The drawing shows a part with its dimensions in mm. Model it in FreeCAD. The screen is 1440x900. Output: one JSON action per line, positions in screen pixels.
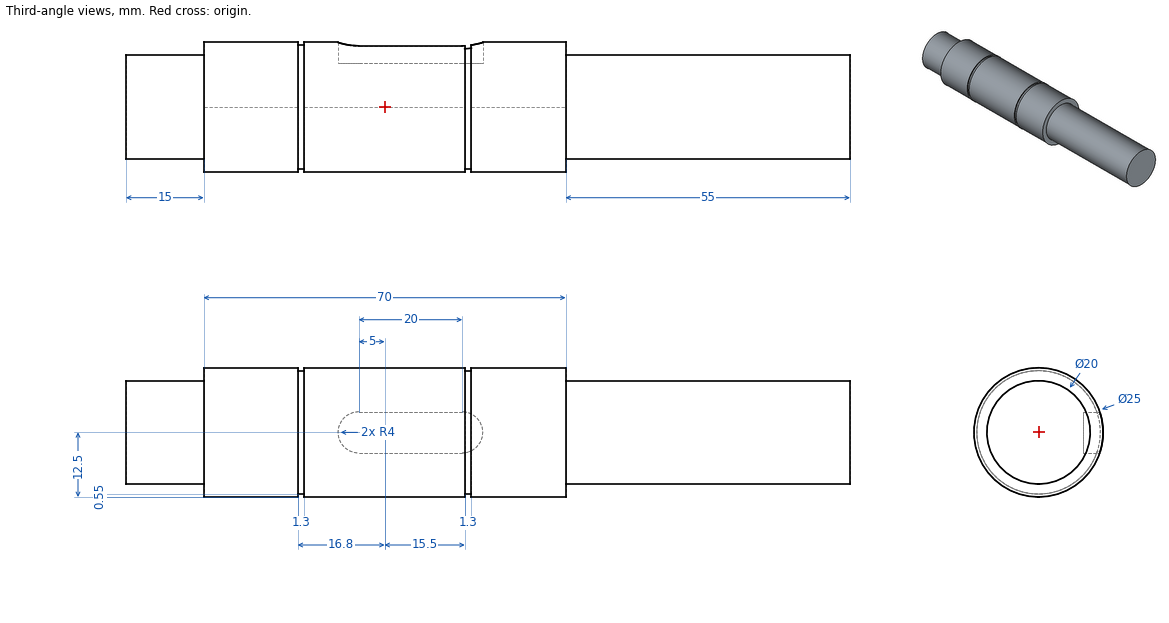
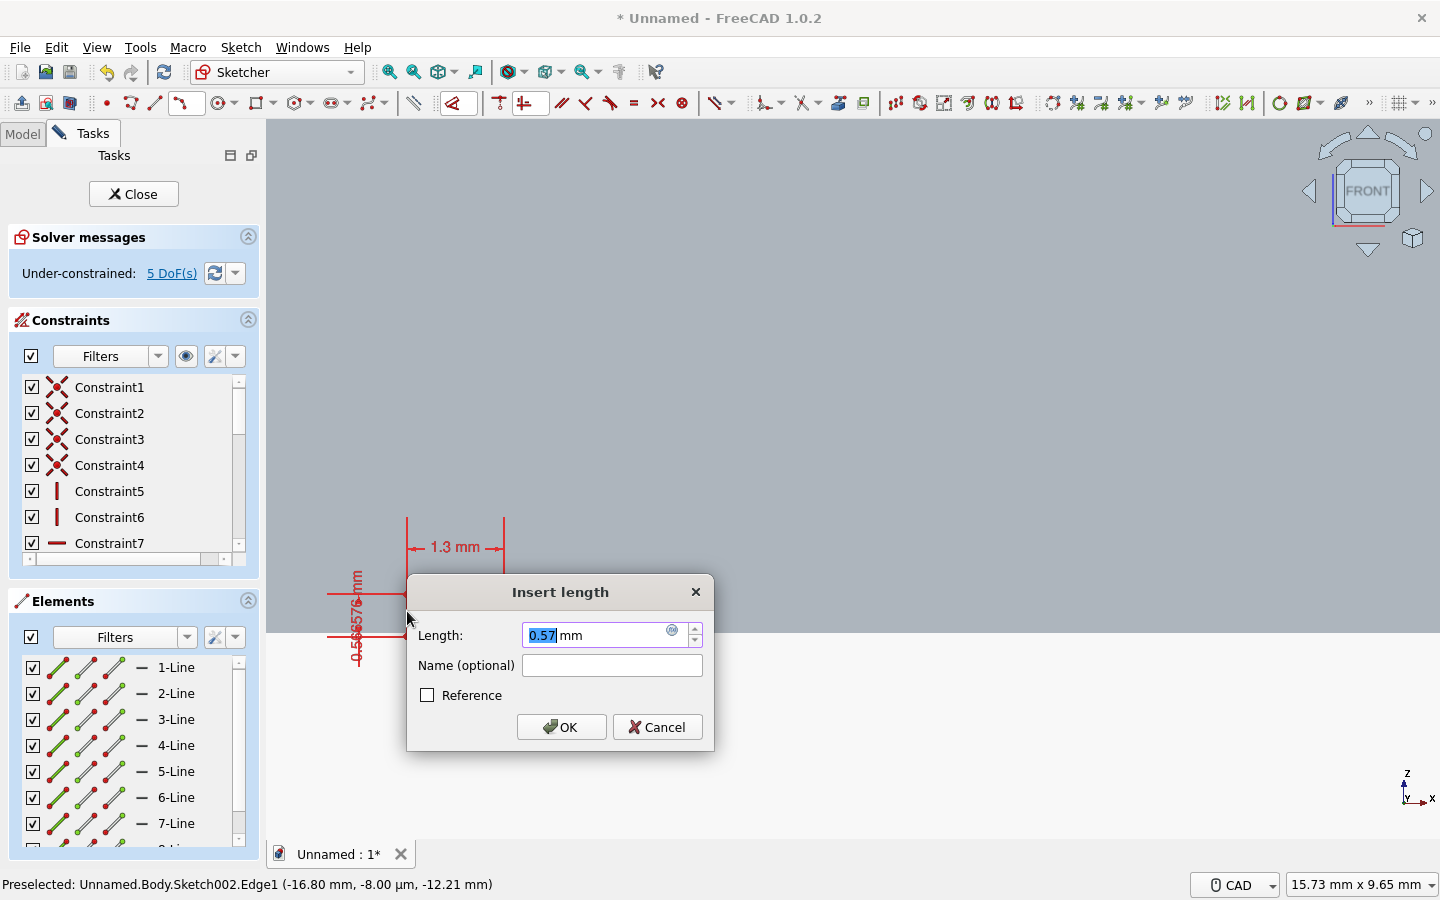
{"action": "type", "text": "0.55"}
{"action": "key", "text": "Return"}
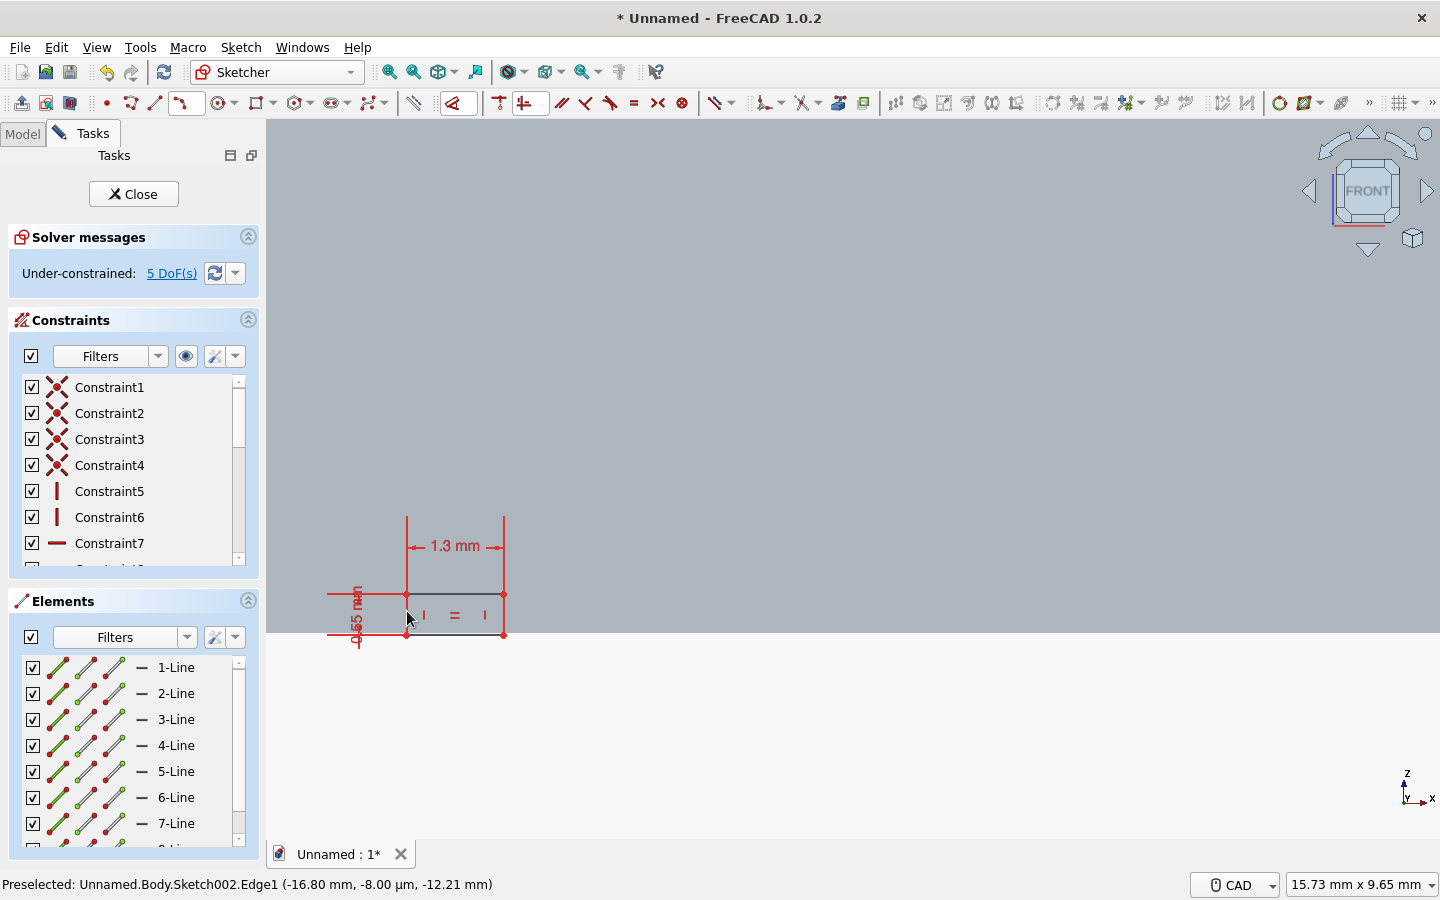
{"action": "scroll", "coordinate": [407, 613], "scroll_direction": "down", "scroll_amount": 6}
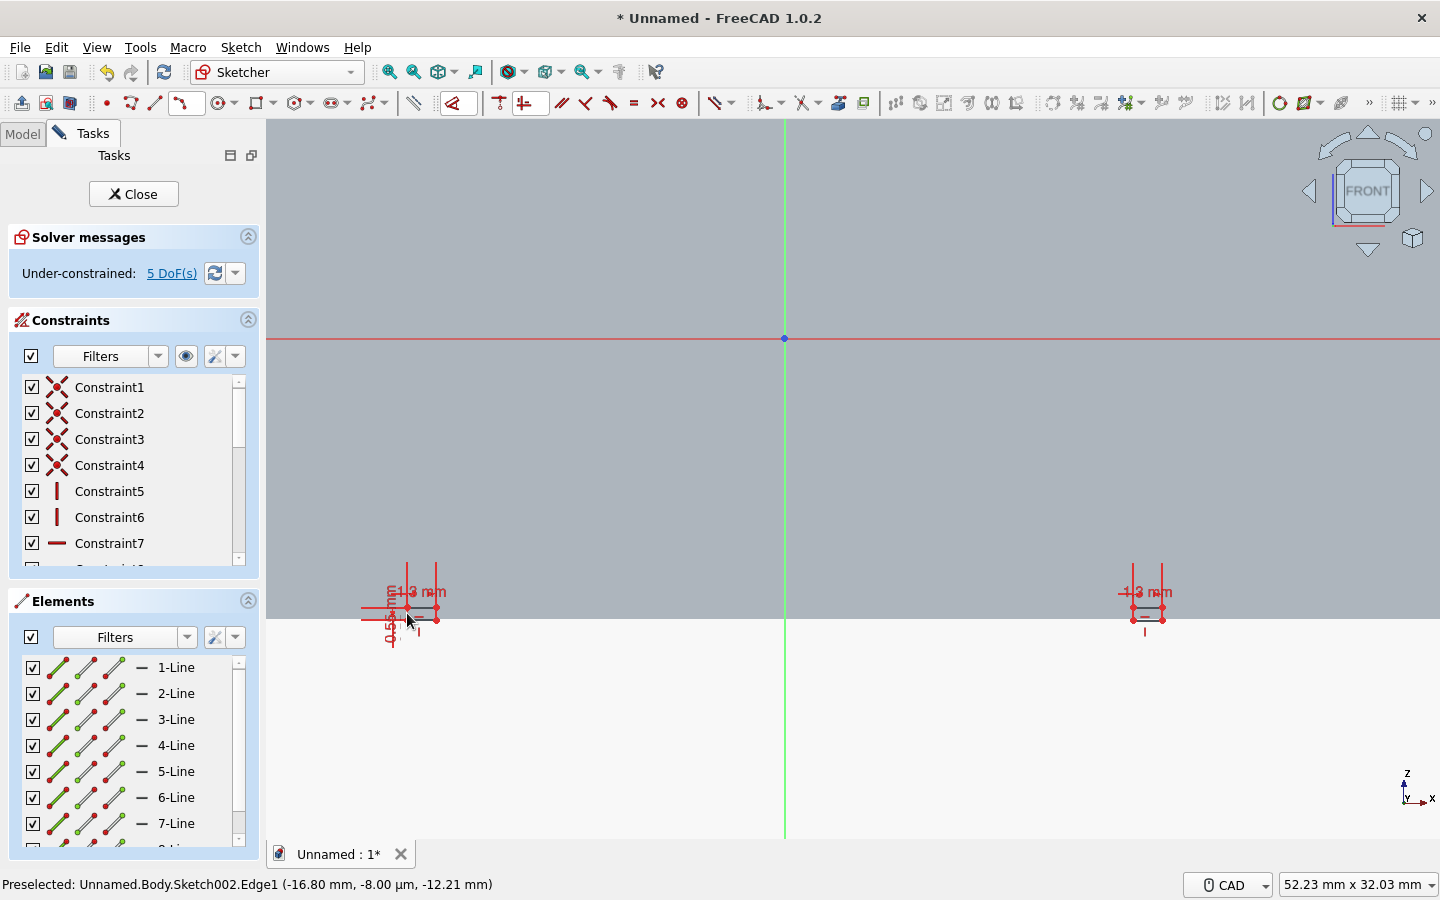
{"action": "scroll", "coordinate": [1133, 612], "scroll_direction": "up", "scroll_amount": 7}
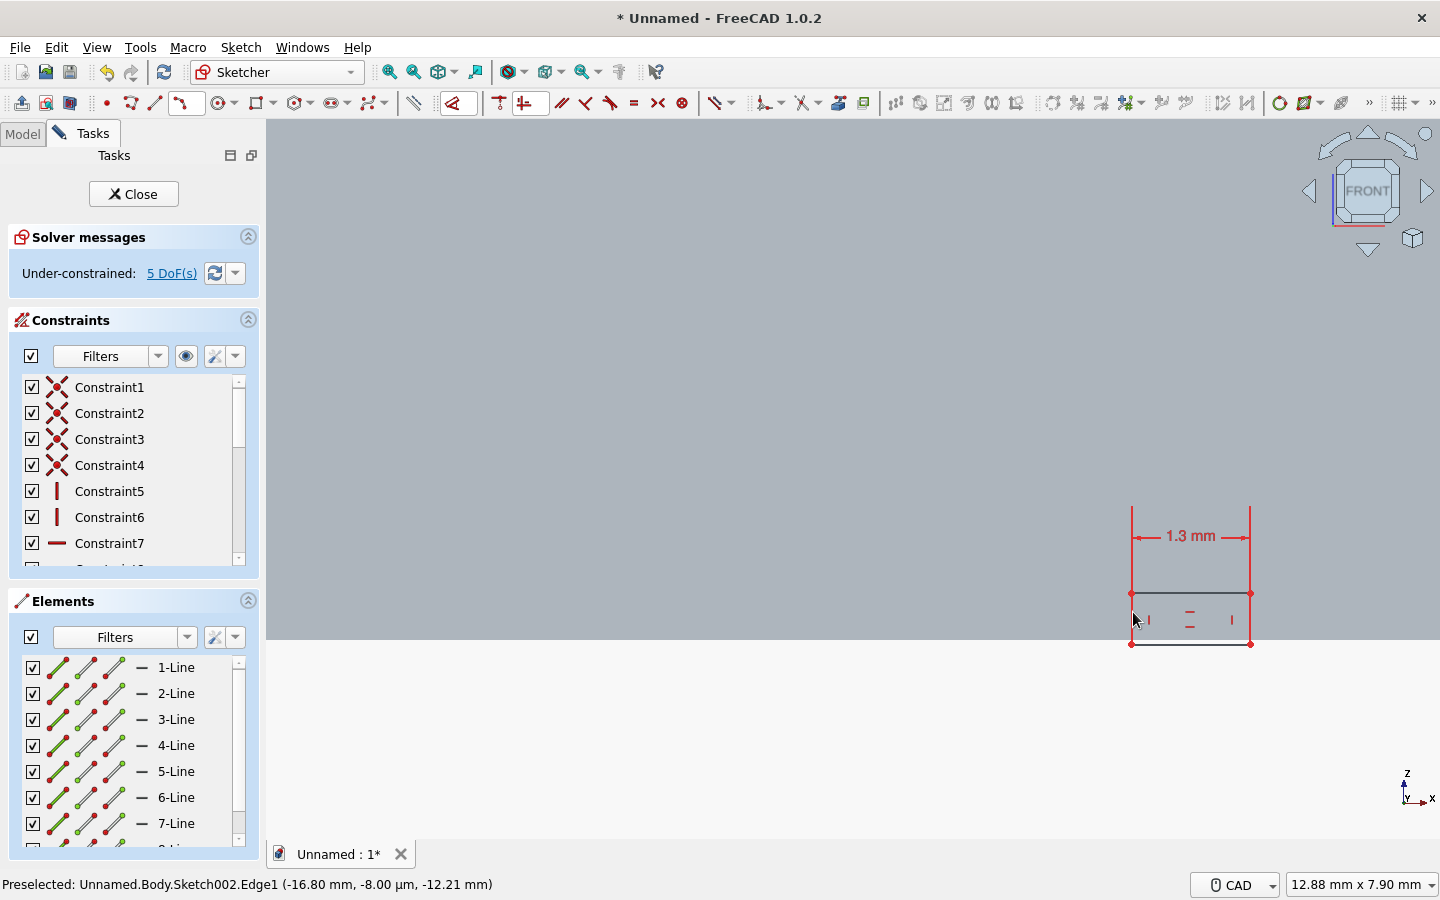
{"action": "left_click", "coordinate": [1132, 609]}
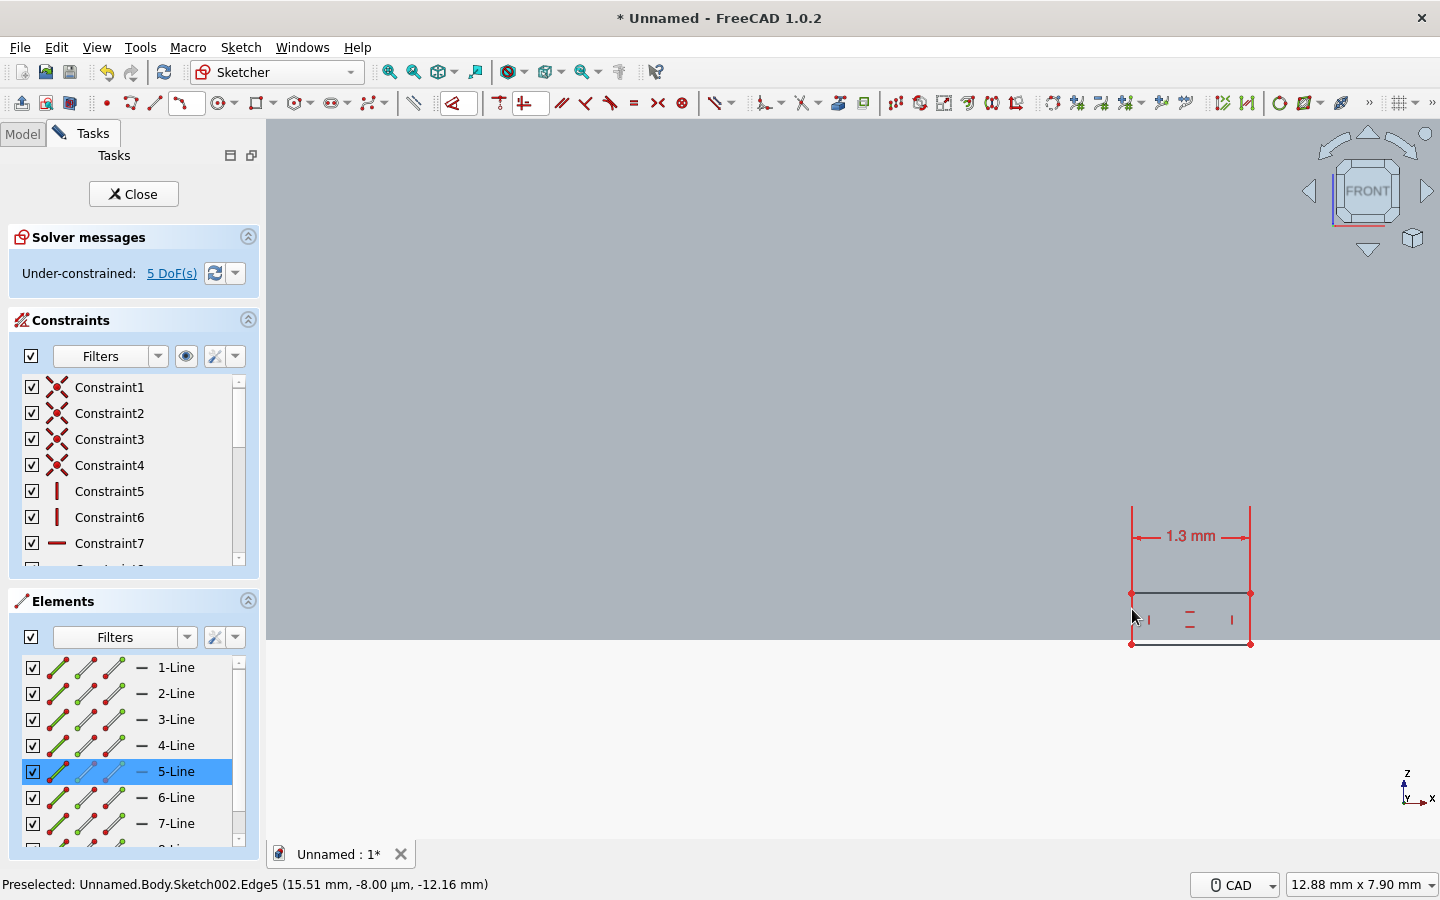
{"action": "left_click", "coordinate": [472, 104]}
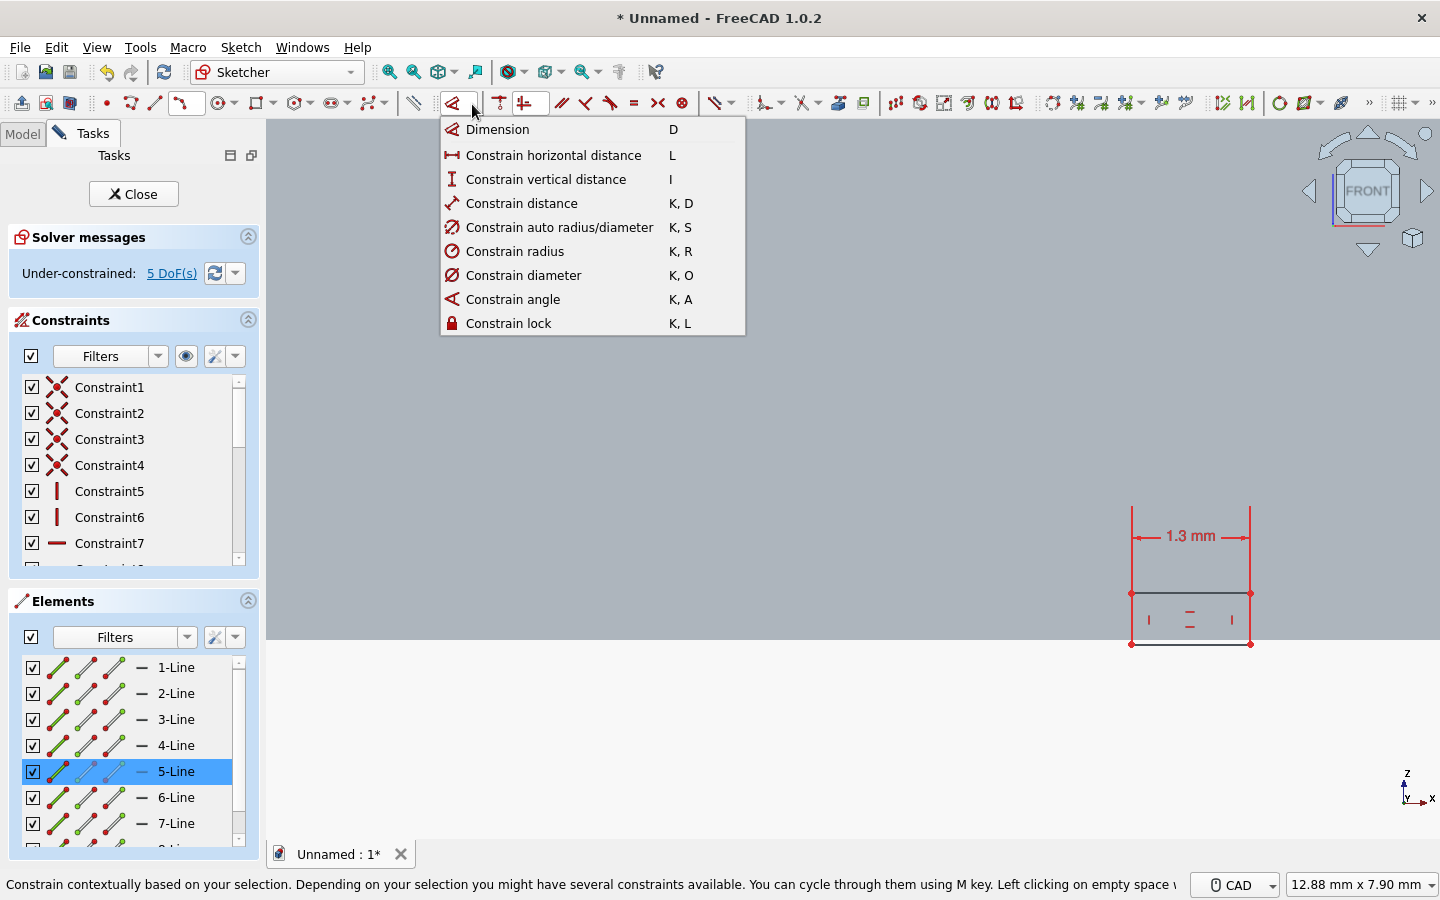
{"action": "left_click", "coordinate": [593, 179]}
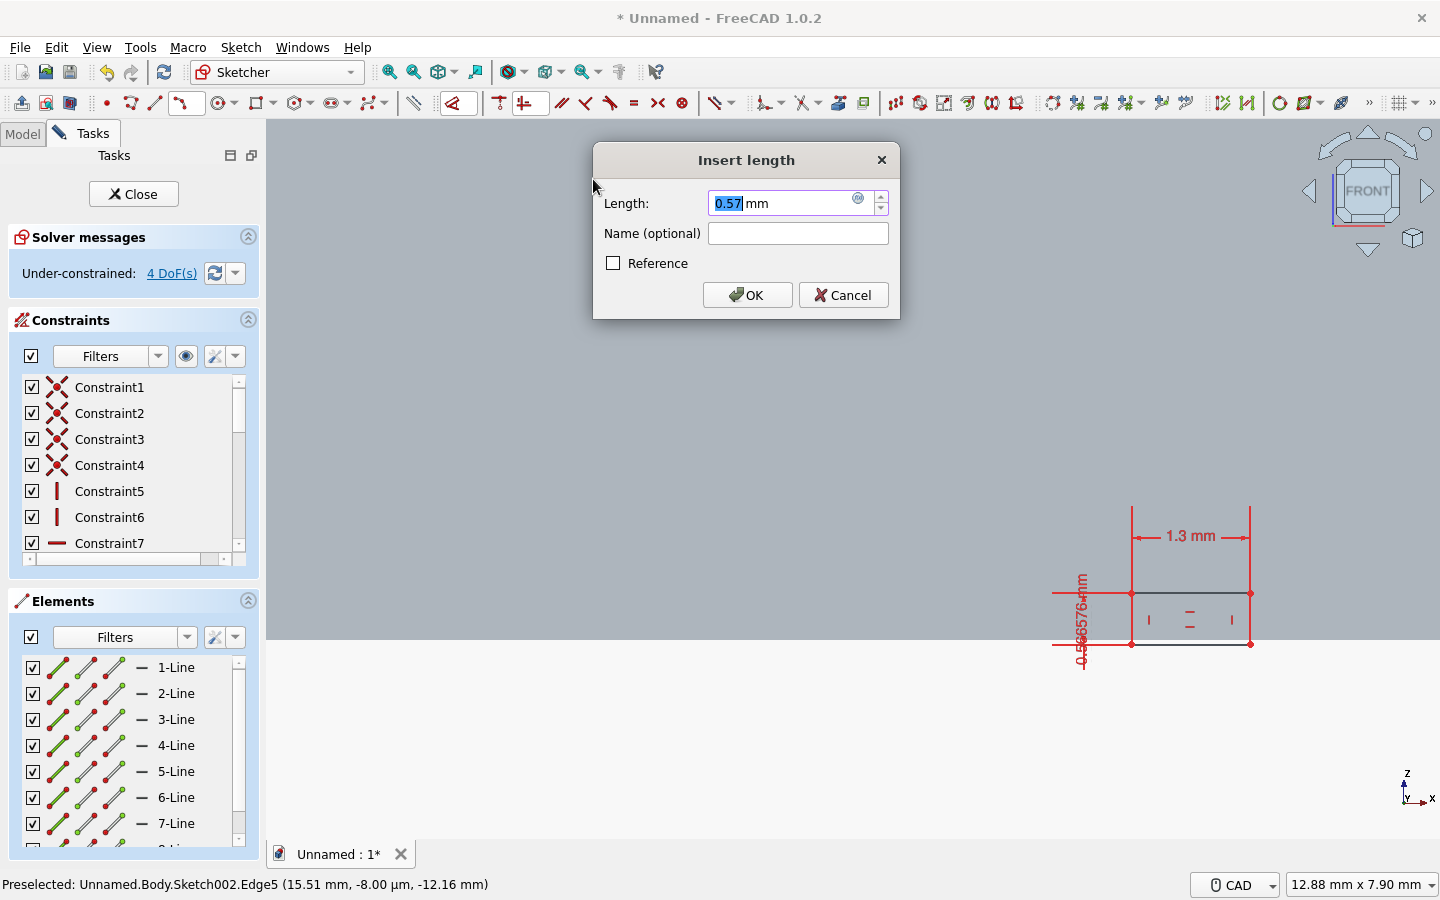
{"action": "type", "text": "0.55"}
{"action": "key", "text": "Return"}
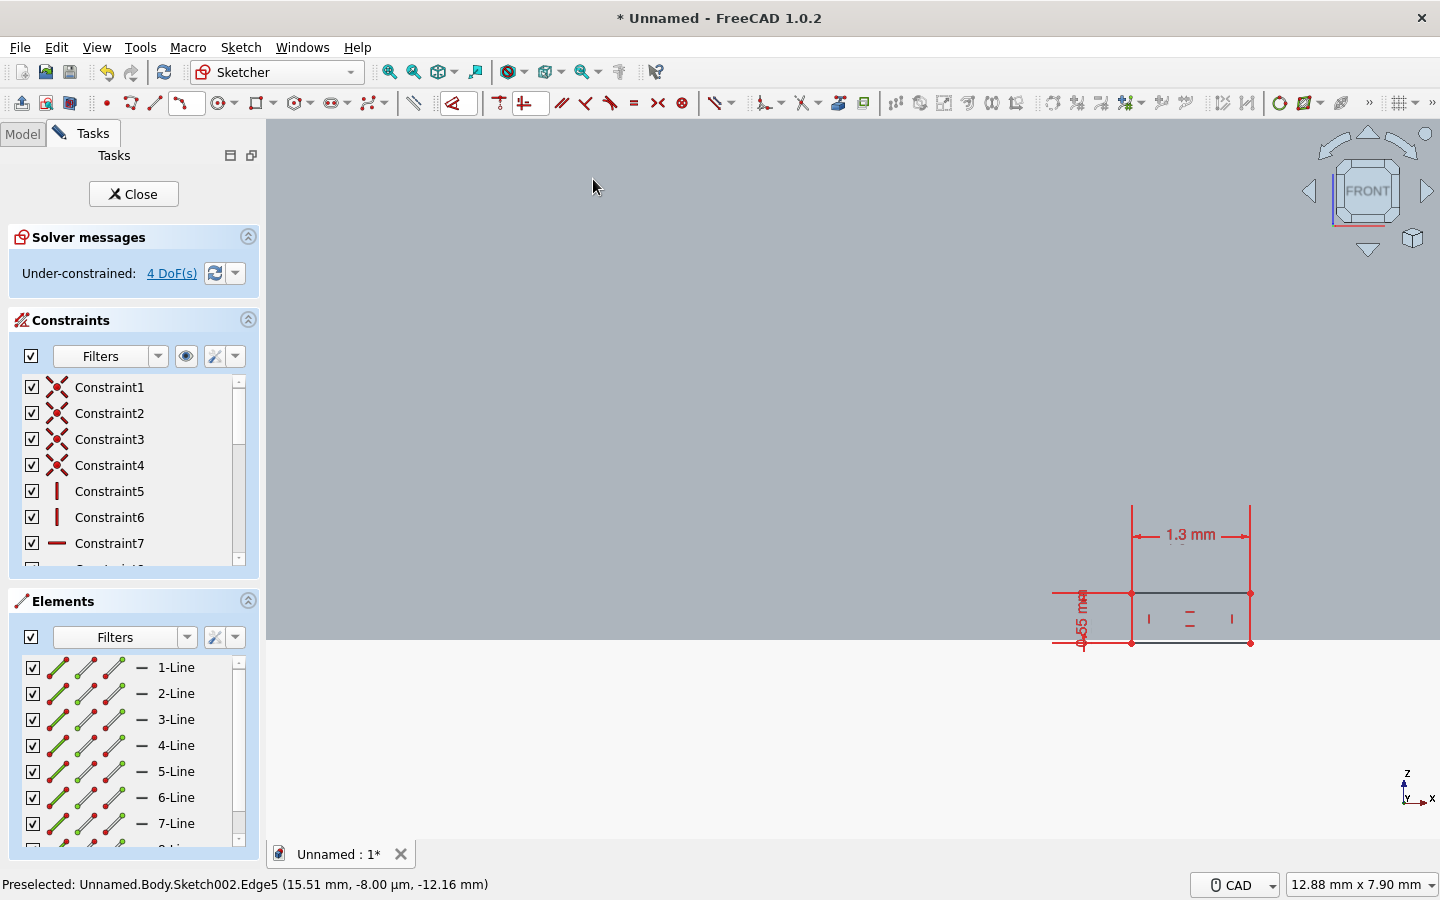
{"action": "scroll", "coordinate": [1133, 612], "scroll_direction": "down", "scroll_amount": 7}